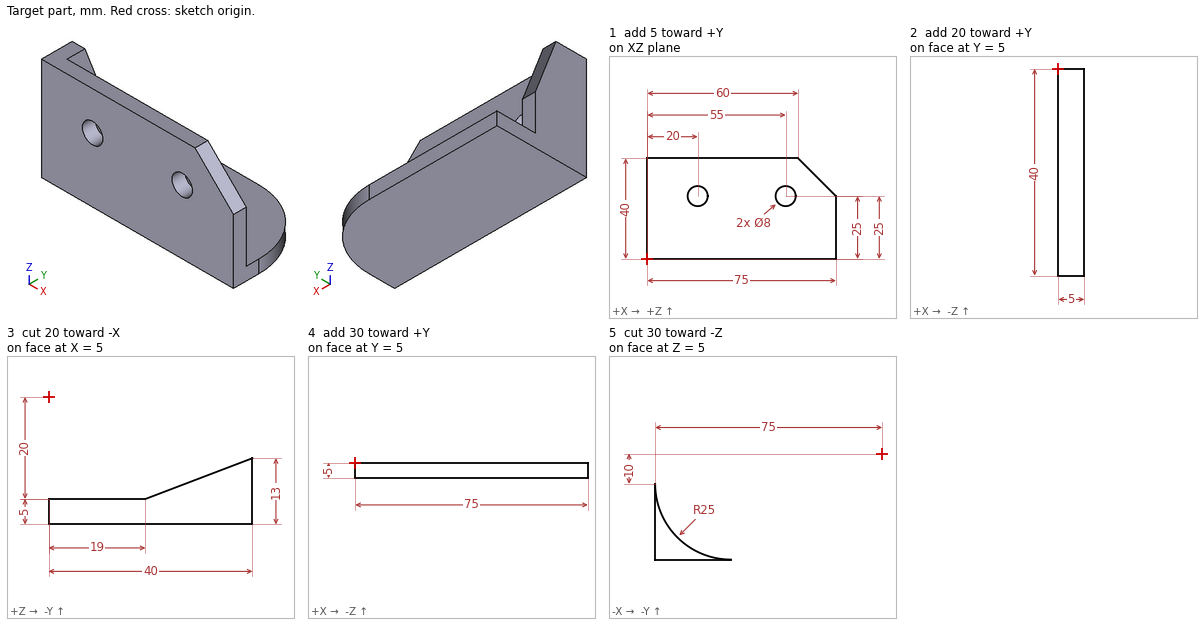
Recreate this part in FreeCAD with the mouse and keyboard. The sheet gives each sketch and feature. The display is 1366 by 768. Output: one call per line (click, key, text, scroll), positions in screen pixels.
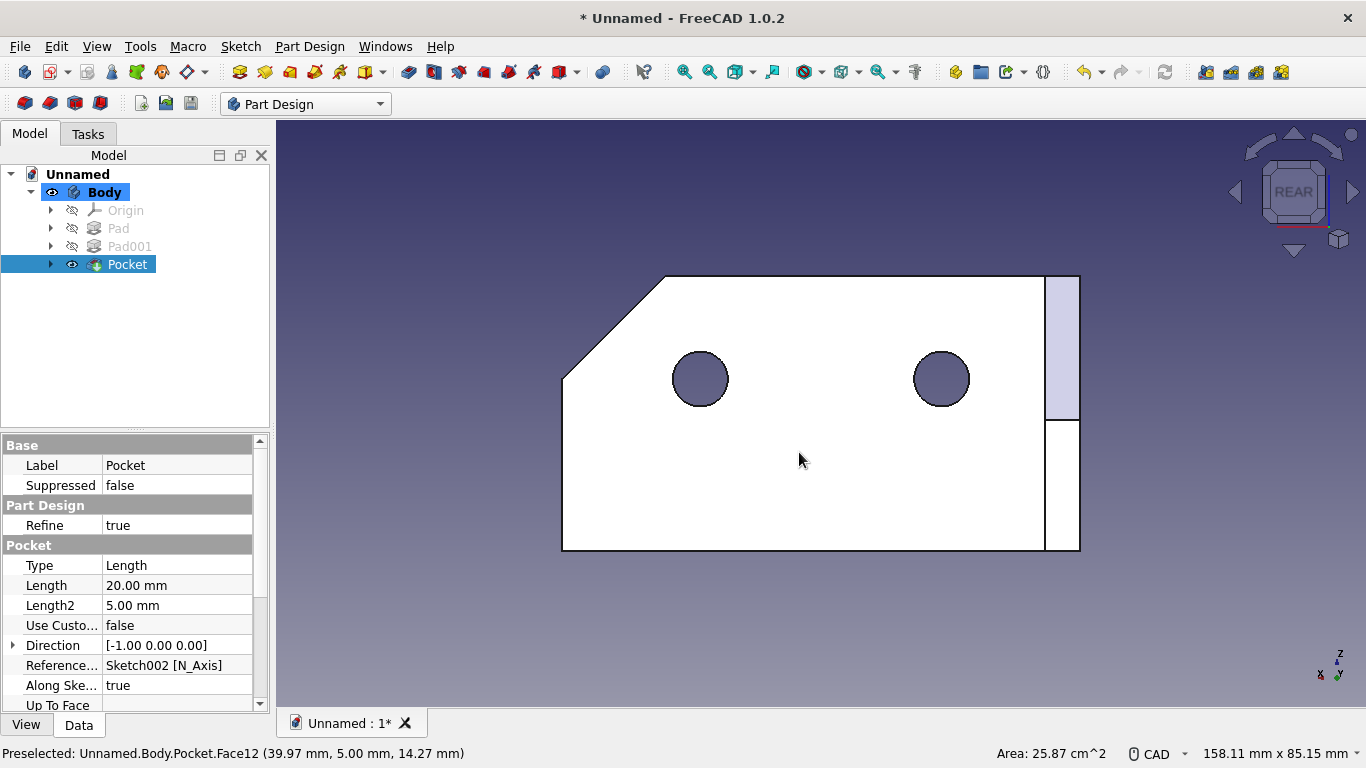
click(50, 72)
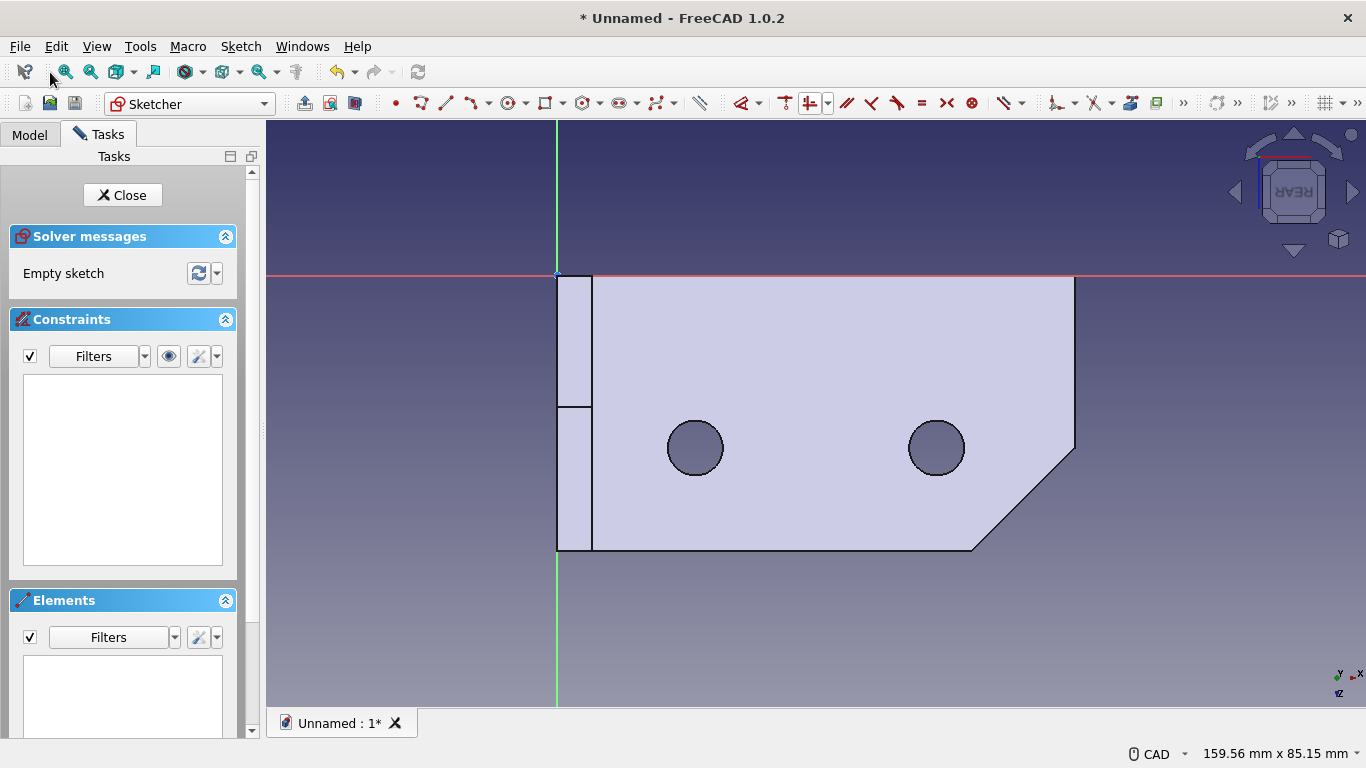
click(544, 104)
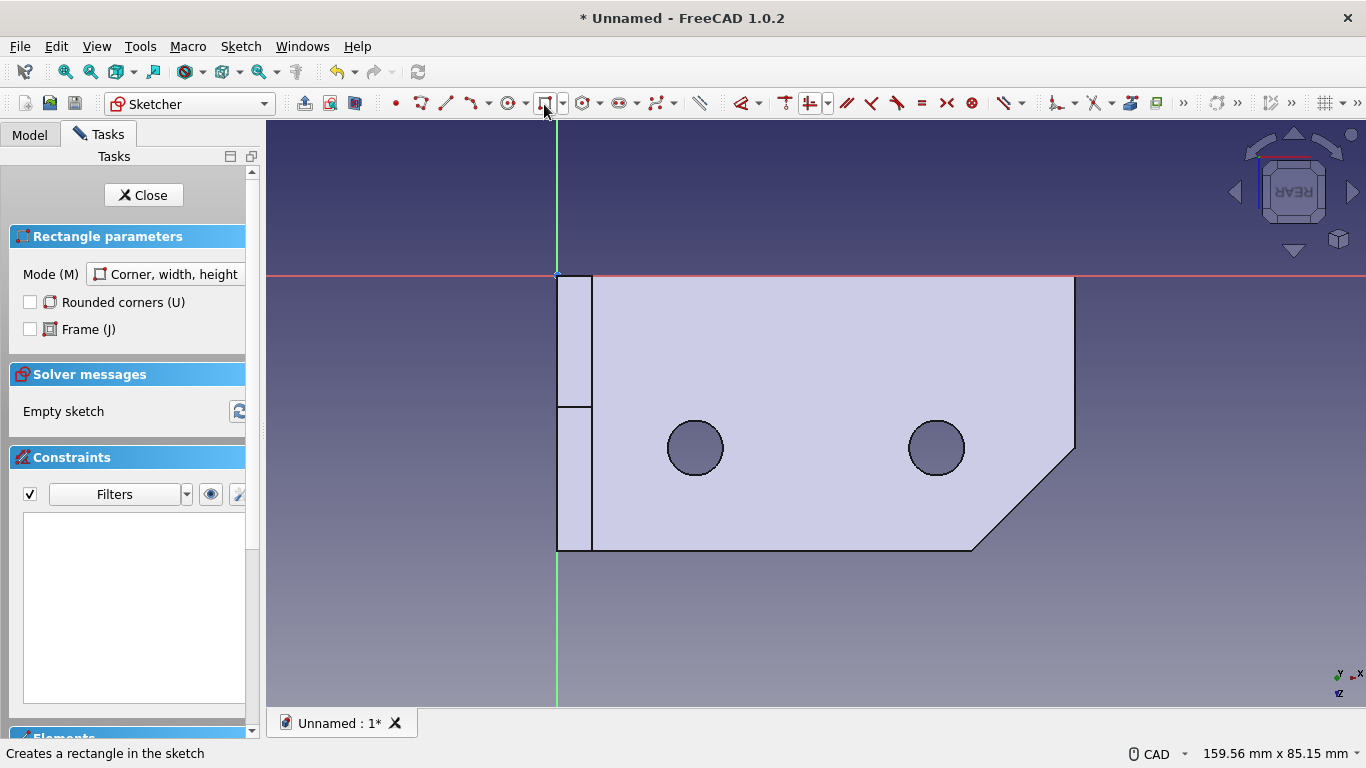
click(557, 276)
click(1075, 310)
key(Escape)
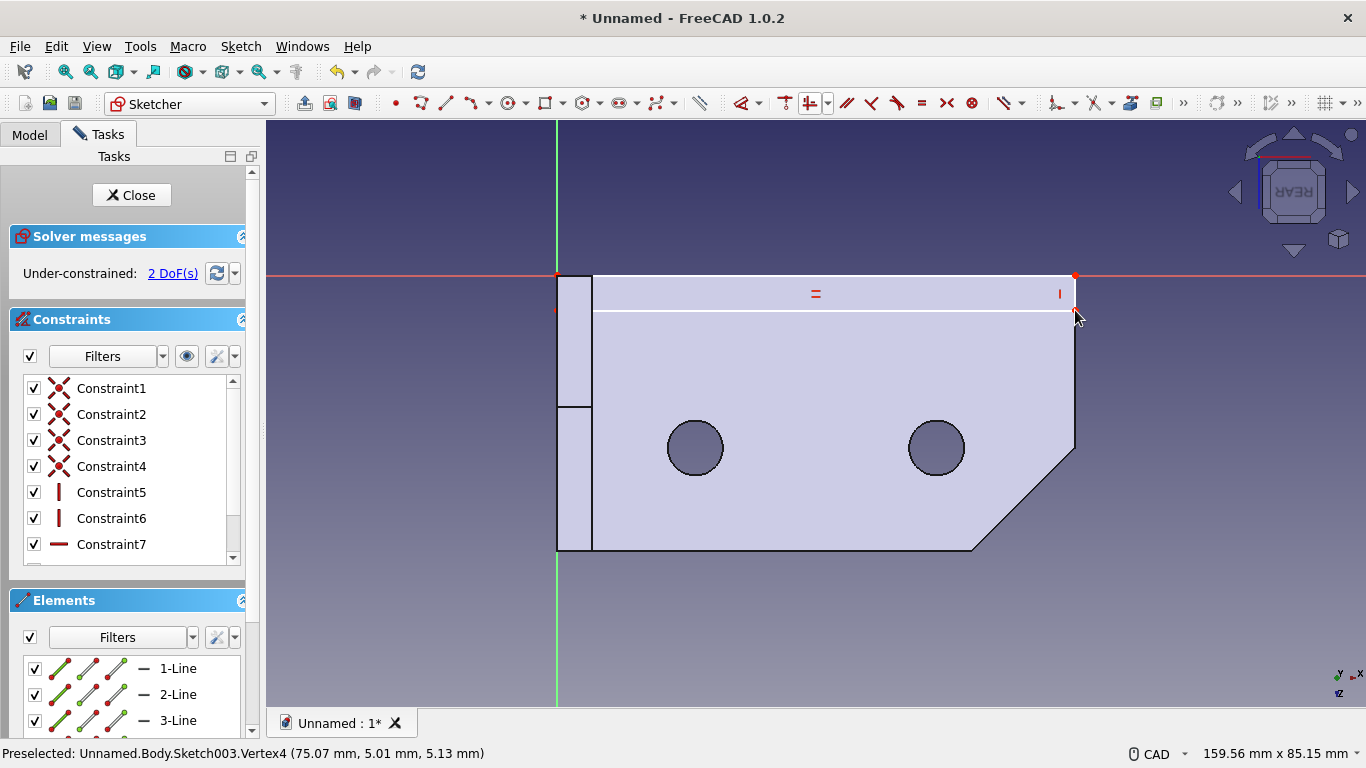
click(740, 104)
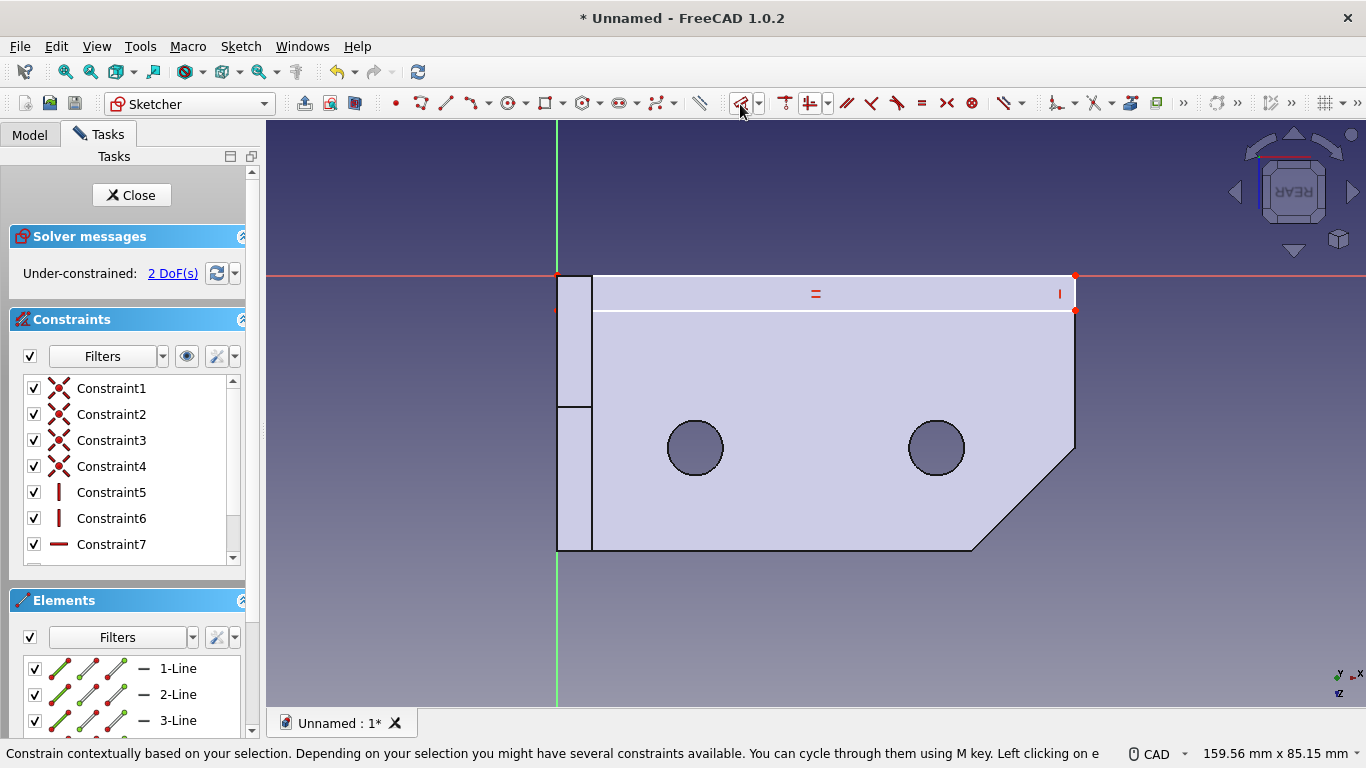
scroll(557, 286, up, 2)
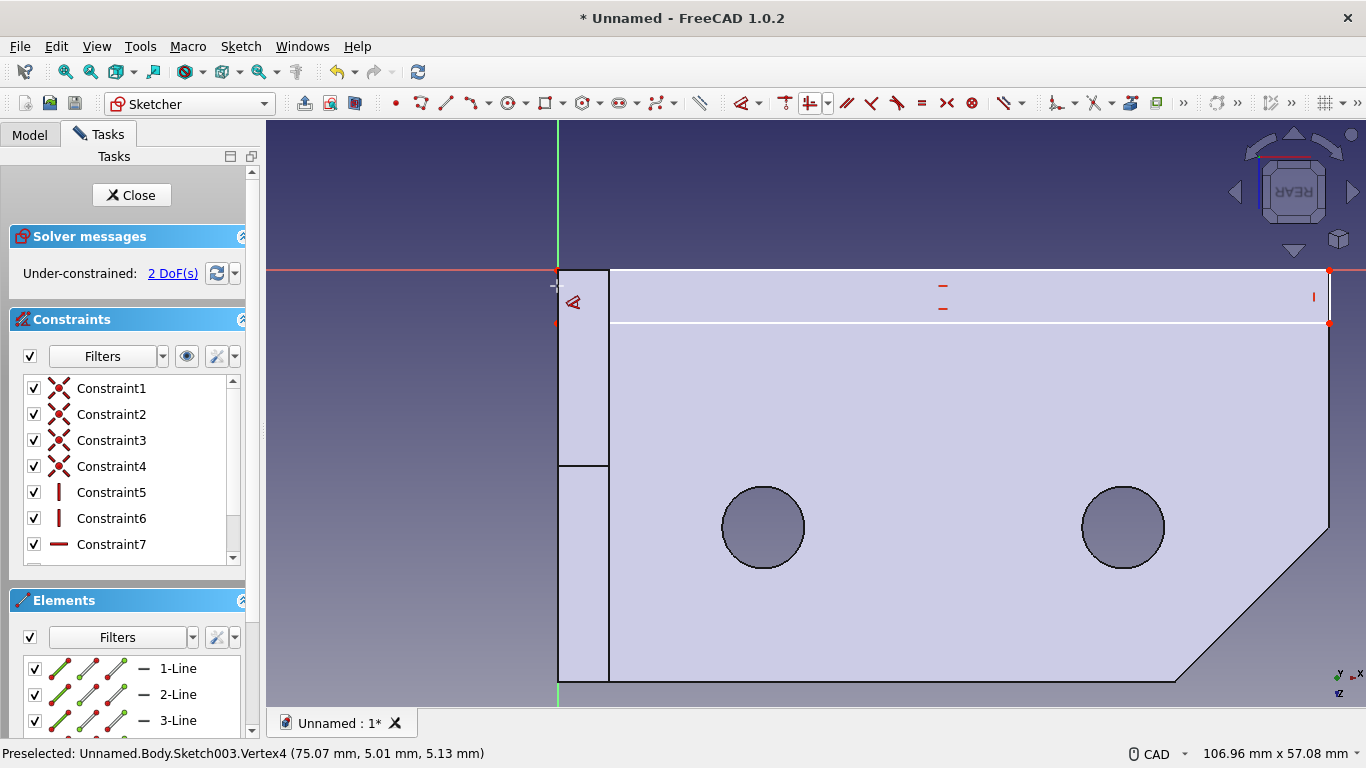
click(558, 286)
click(524, 297)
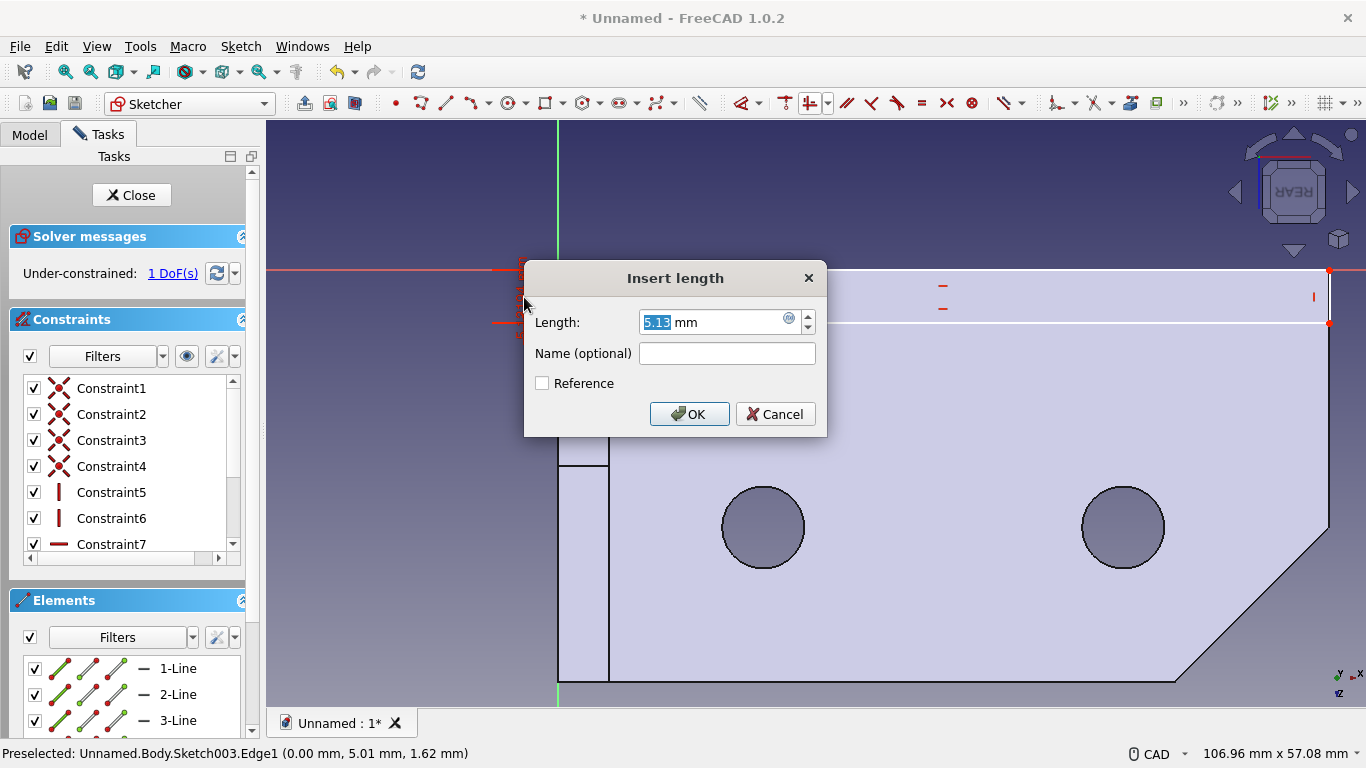
text(5)
key(Return)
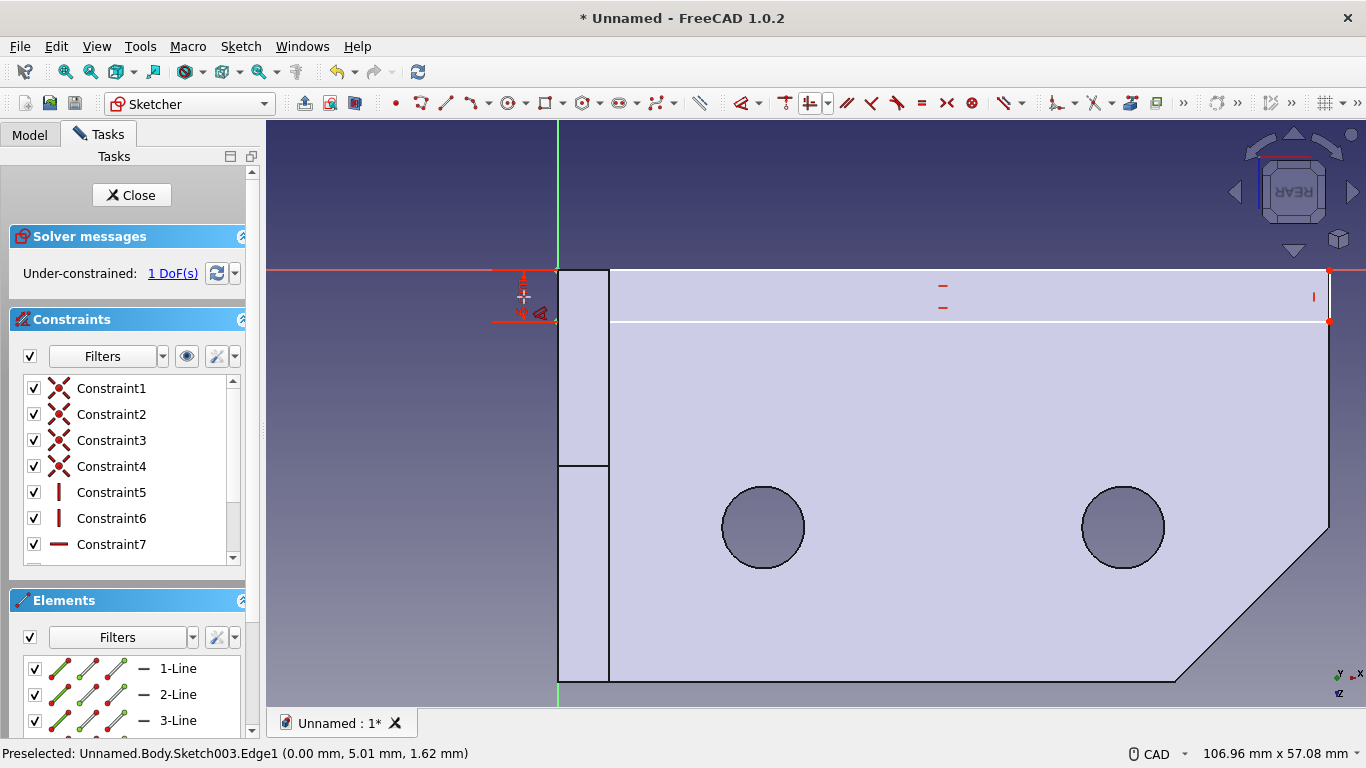
click(789, 322)
click(879, 356)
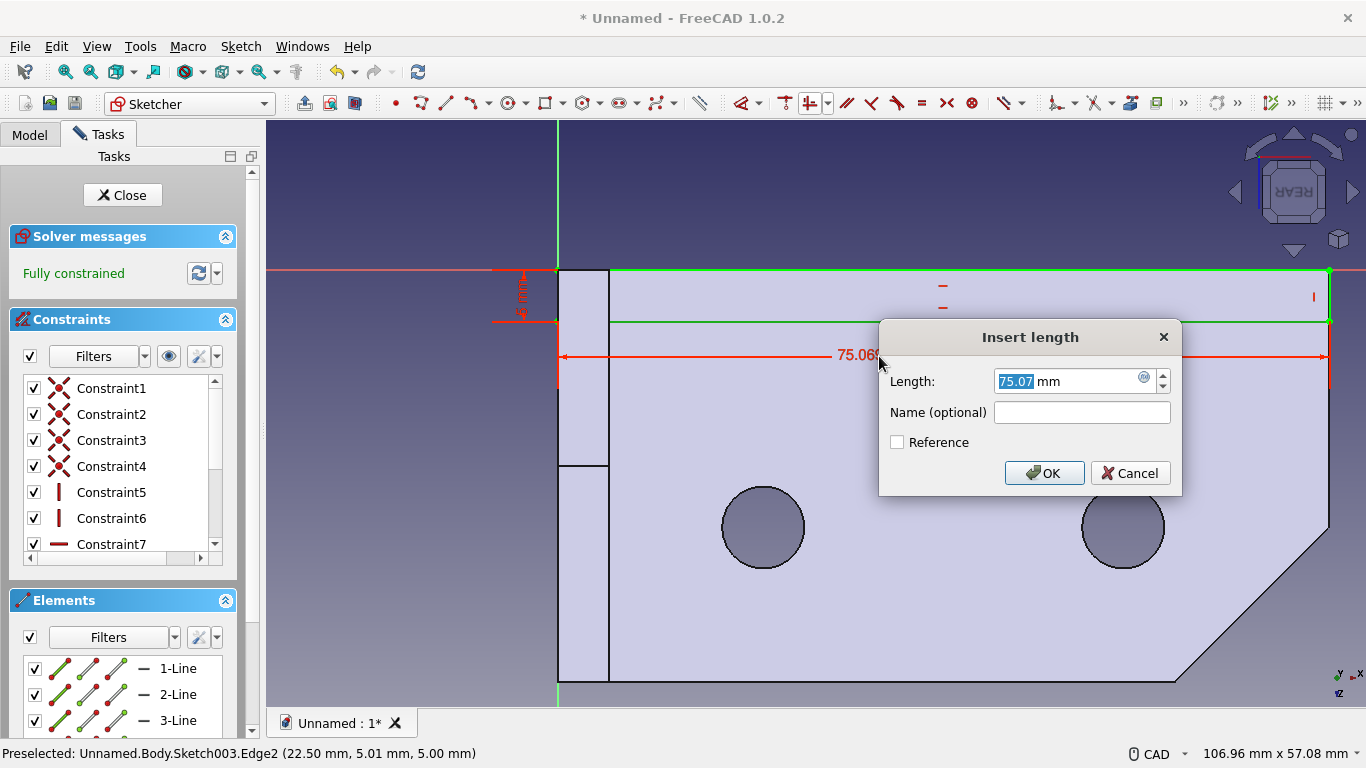
text(75)
key(Return)
key(Escape)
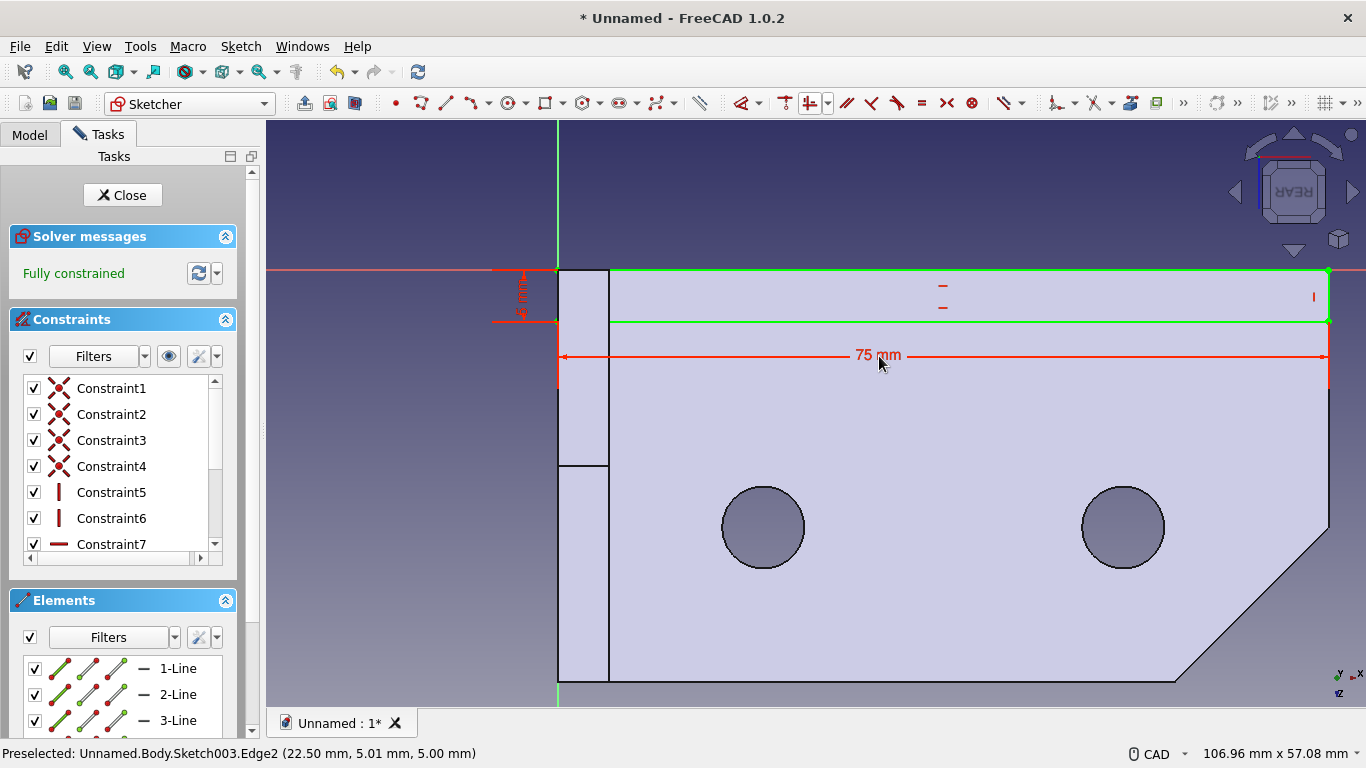
click(123, 195)